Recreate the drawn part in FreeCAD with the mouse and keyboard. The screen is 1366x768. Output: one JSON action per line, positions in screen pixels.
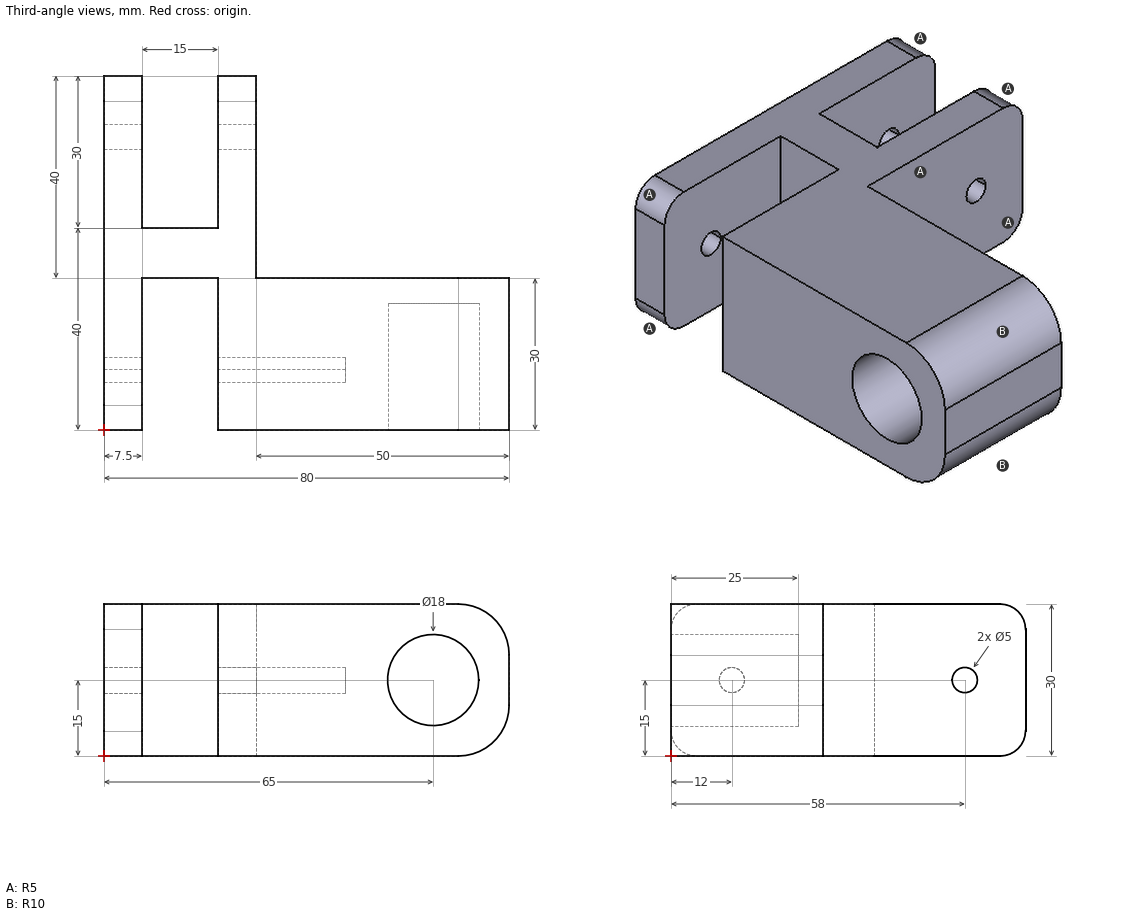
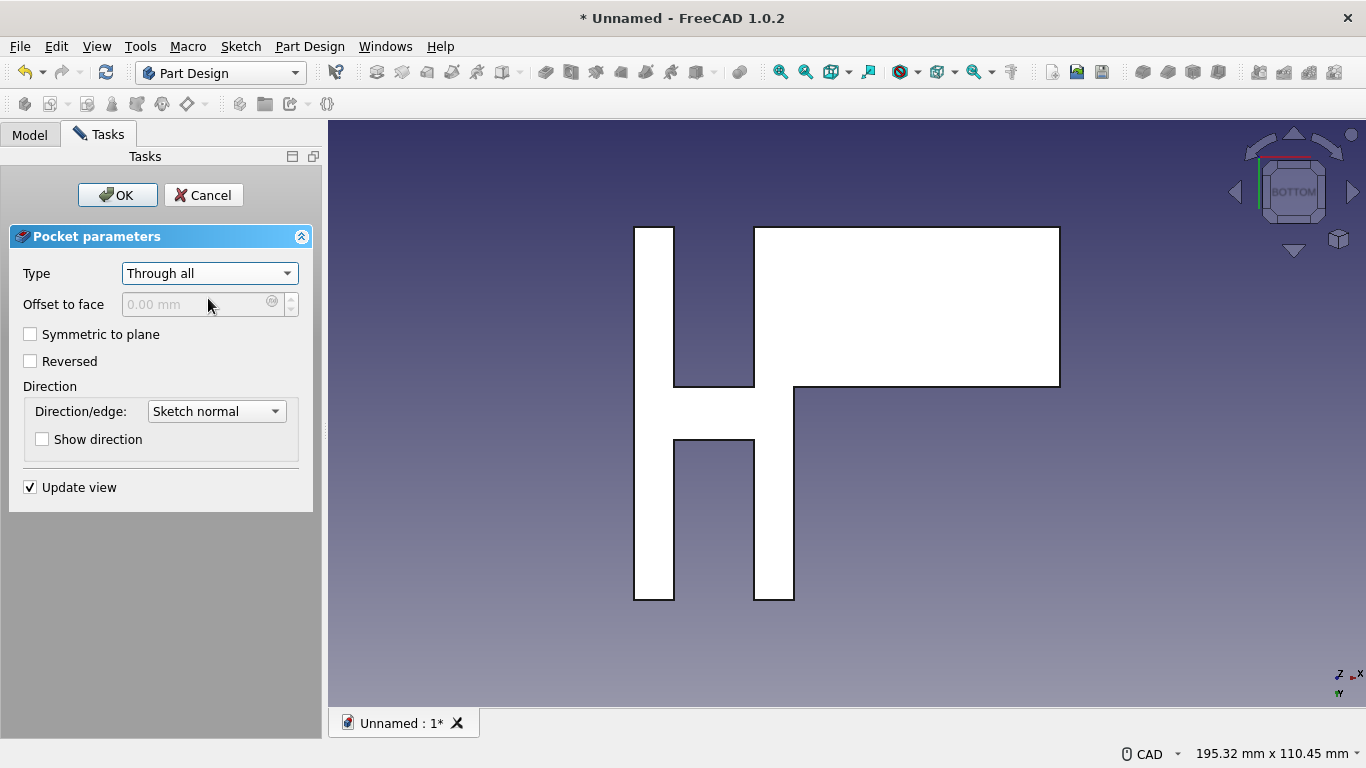
{"action": "left_click", "coordinate": [118, 195]}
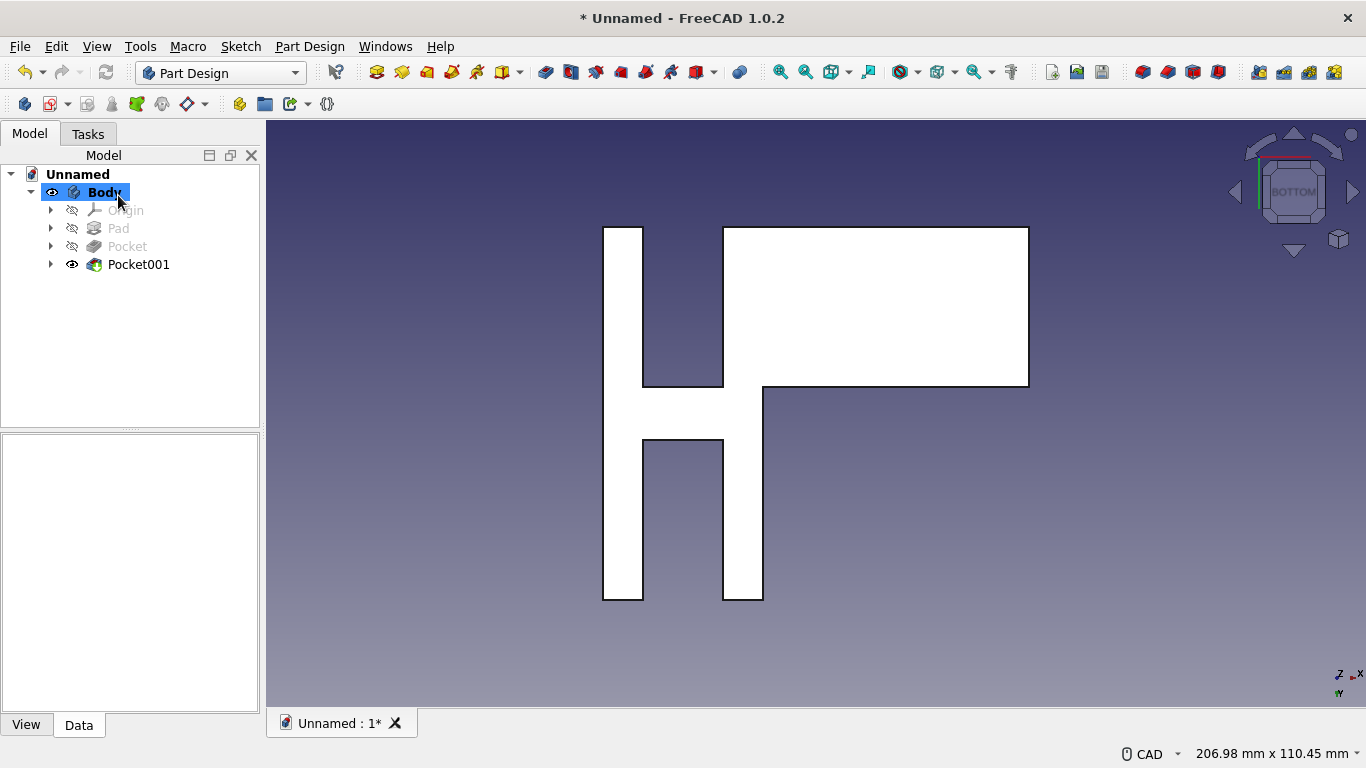
{"action": "left_click", "coordinate": [51, 210]}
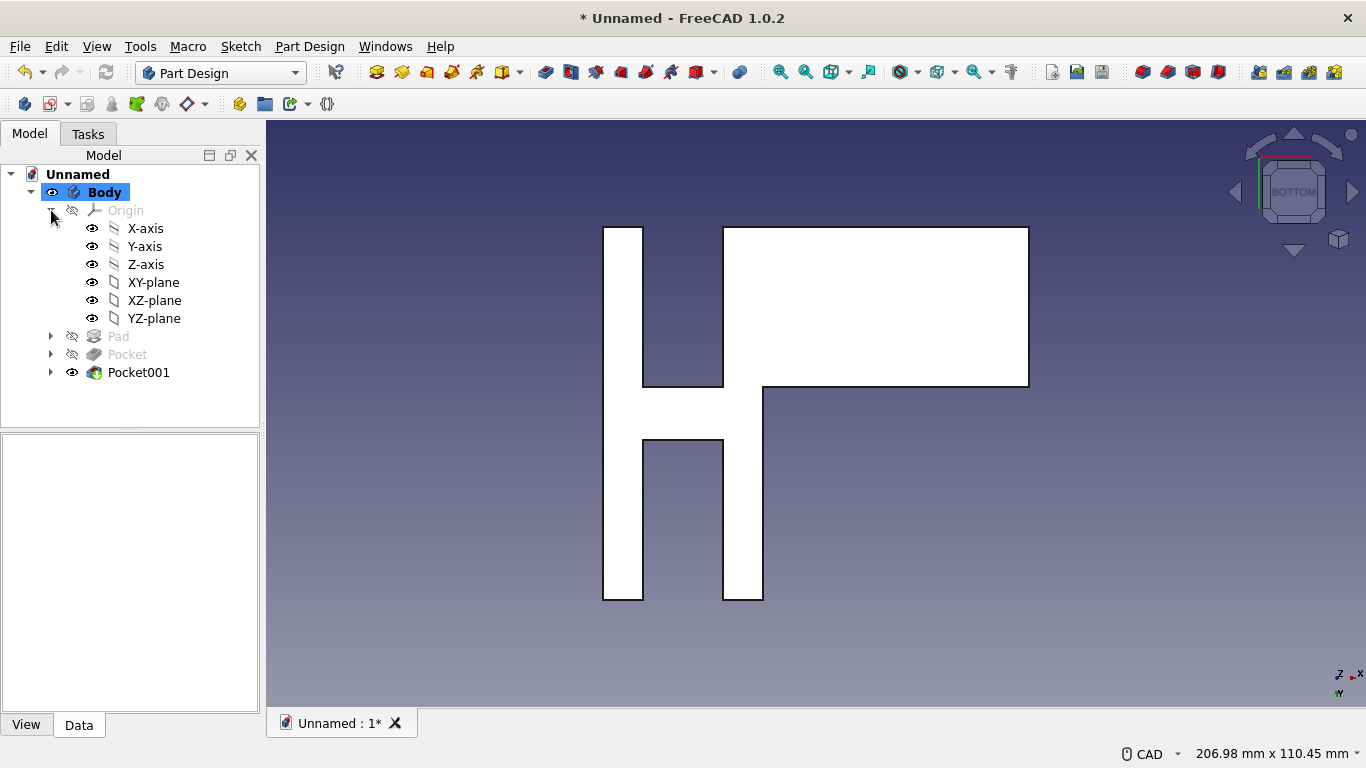
{"action": "left_click", "coordinate": [137, 318]}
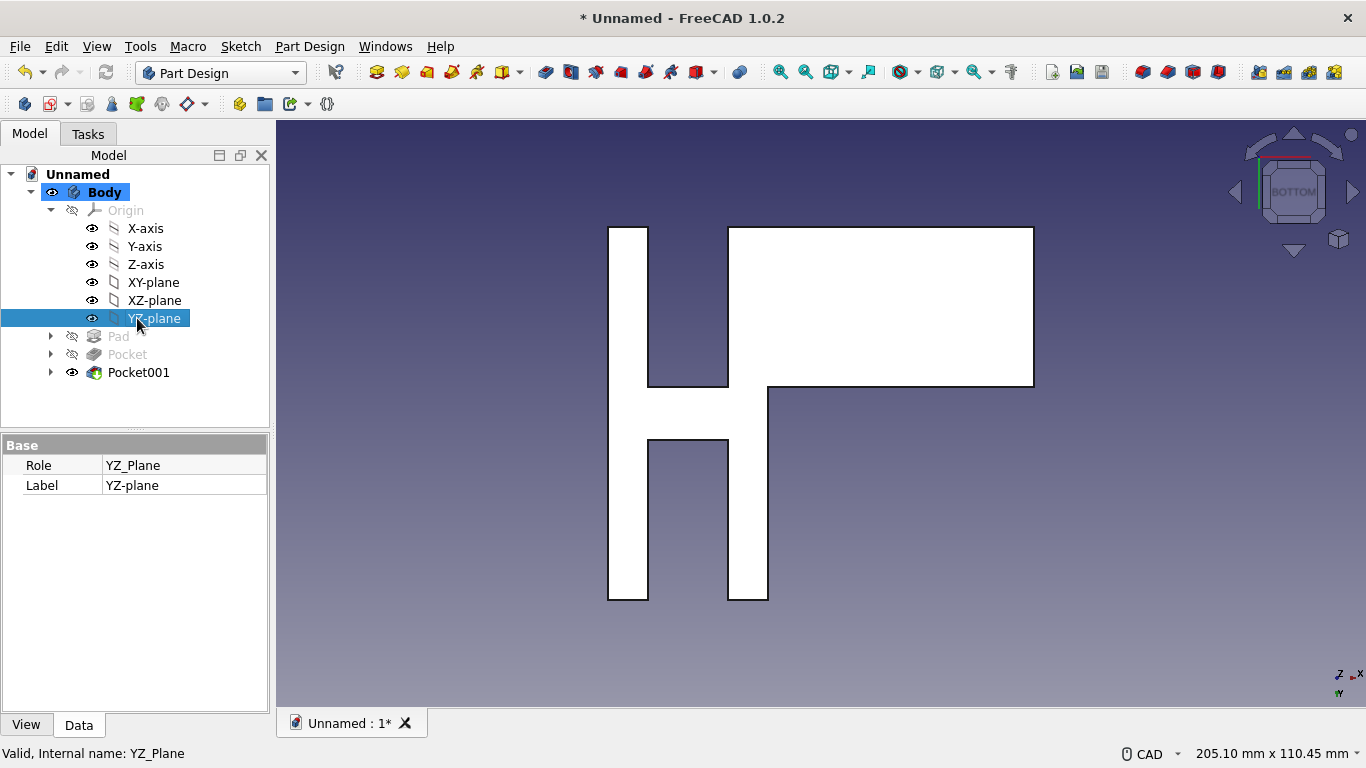
{"action": "left_click", "coordinate": [186, 104]}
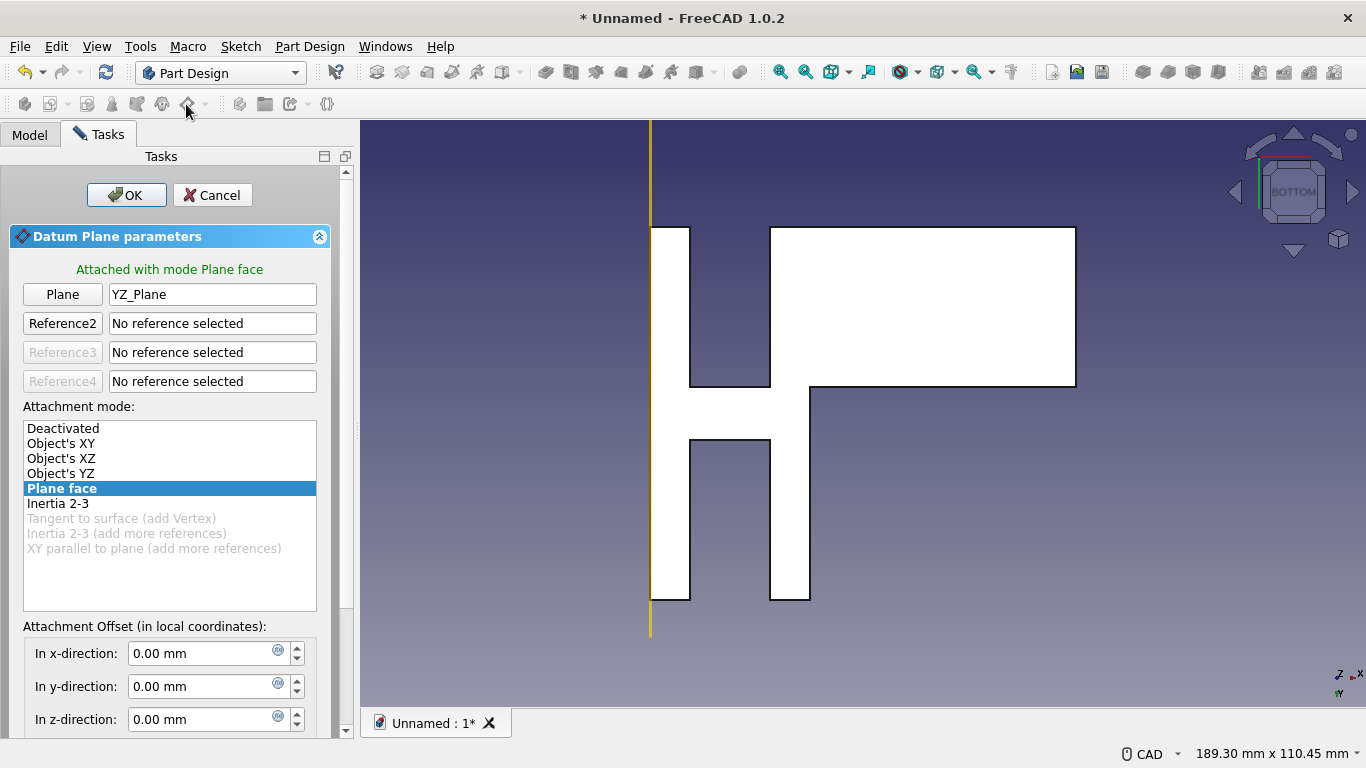
{"action": "triple_click", "coordinate": [210, 720]}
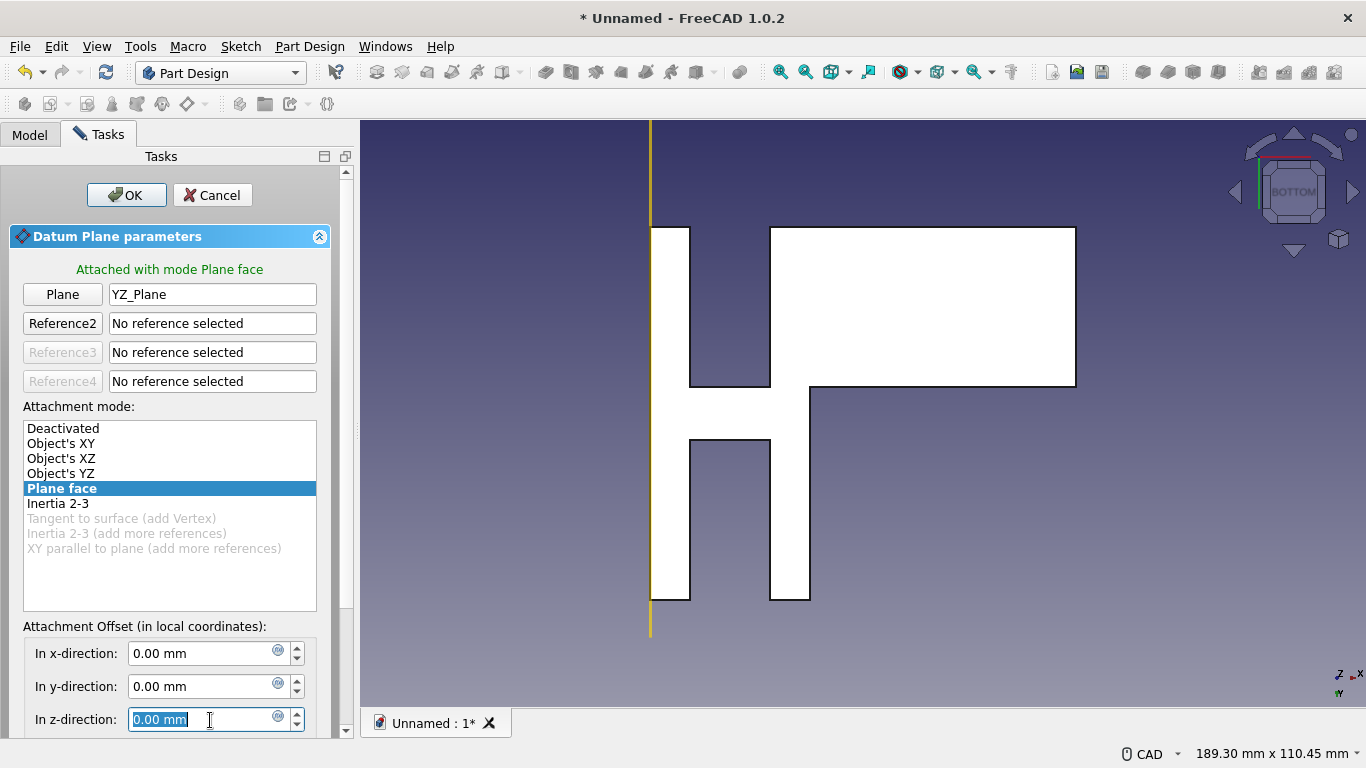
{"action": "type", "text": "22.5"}
{"action": "key", "text": "Tab"}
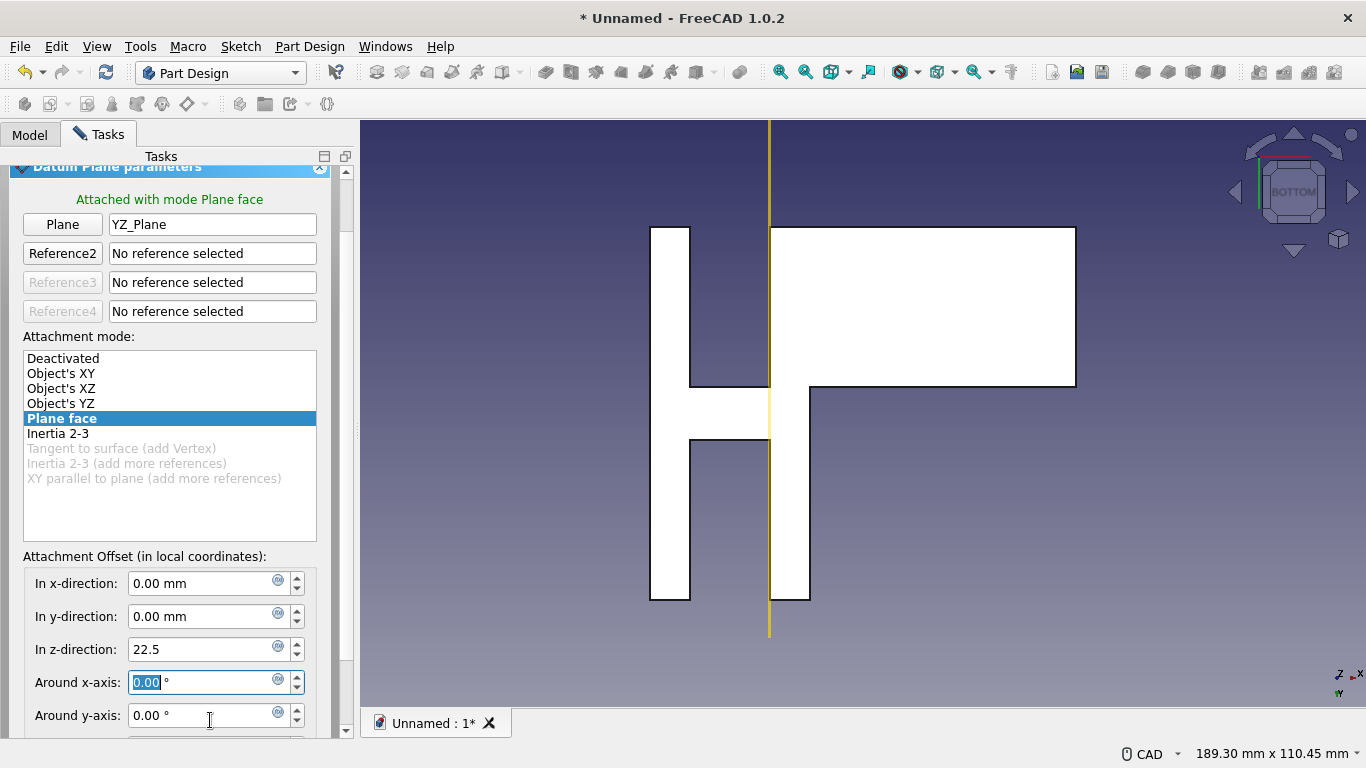
{"action": "scroll", "coordinate": [346, 452], "scroll_direction": "up", "scroll_amount": 2}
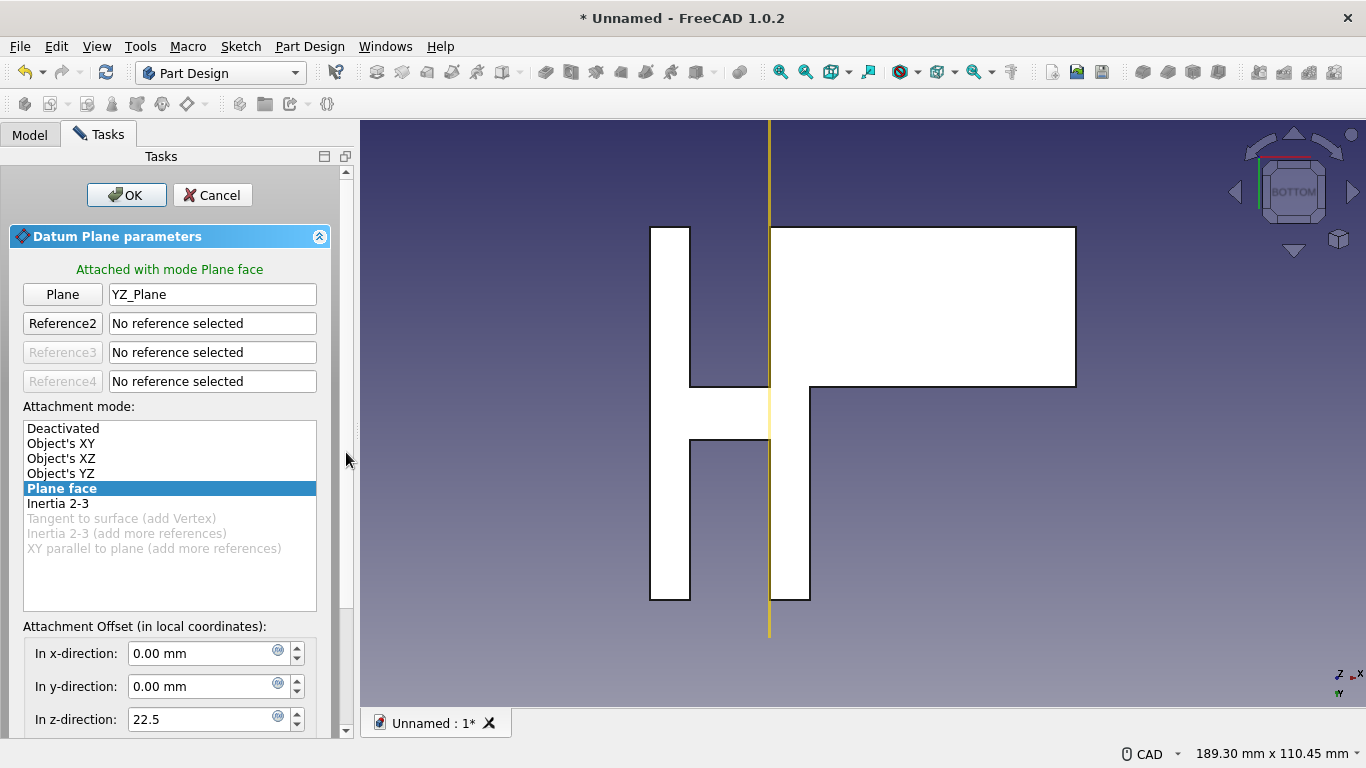
{"action": "left_click", "coordinate": [127, 195]}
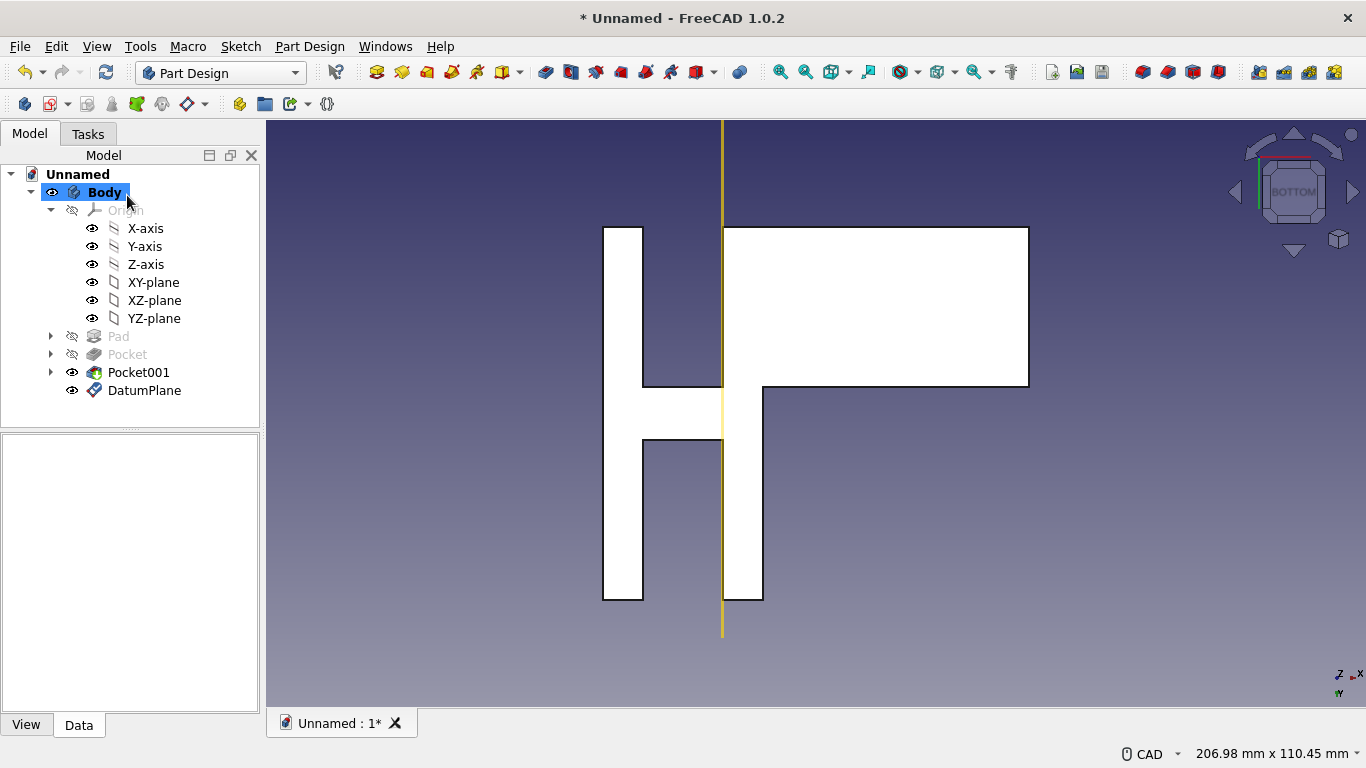
{"action": "left_click", "coordinate": [117, 390]}